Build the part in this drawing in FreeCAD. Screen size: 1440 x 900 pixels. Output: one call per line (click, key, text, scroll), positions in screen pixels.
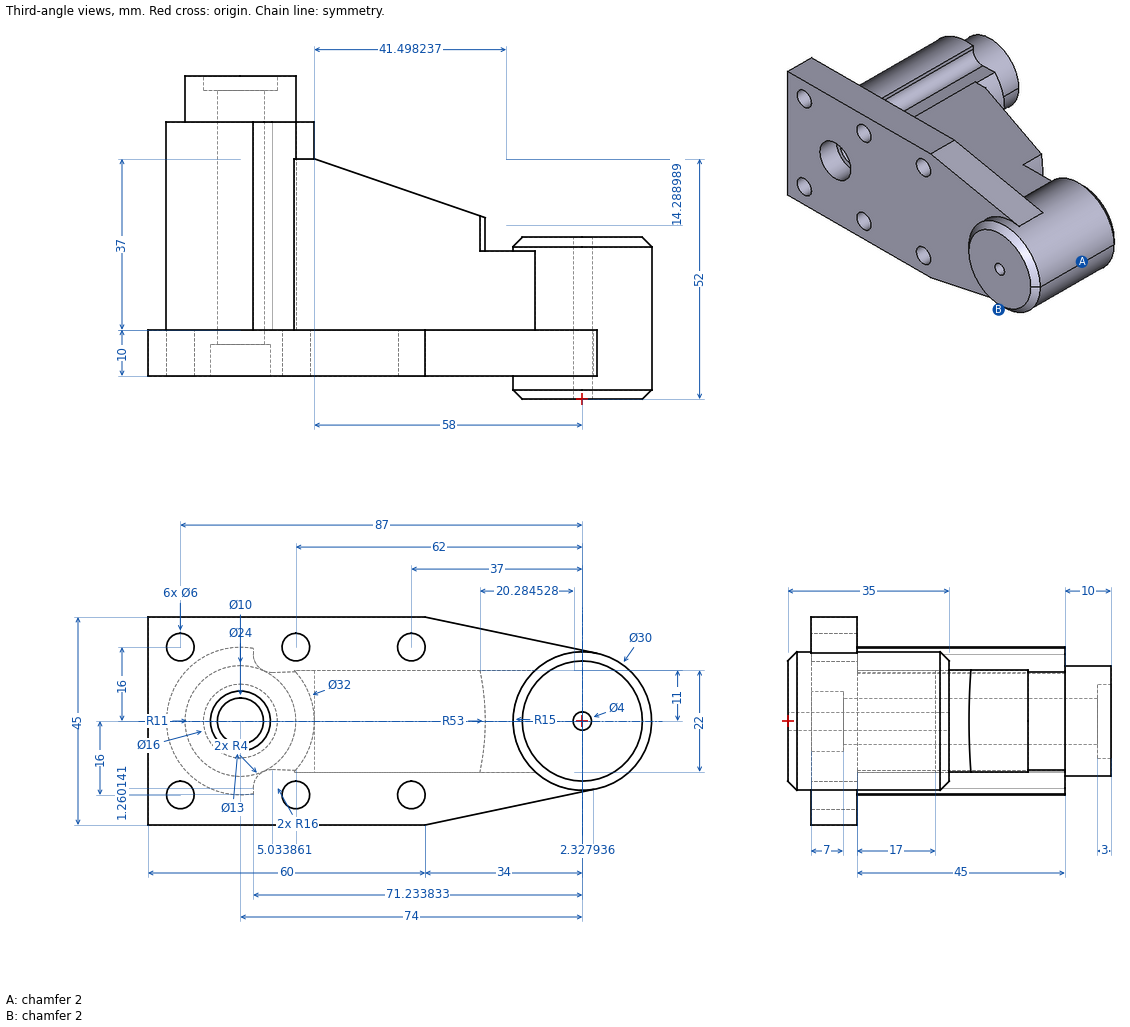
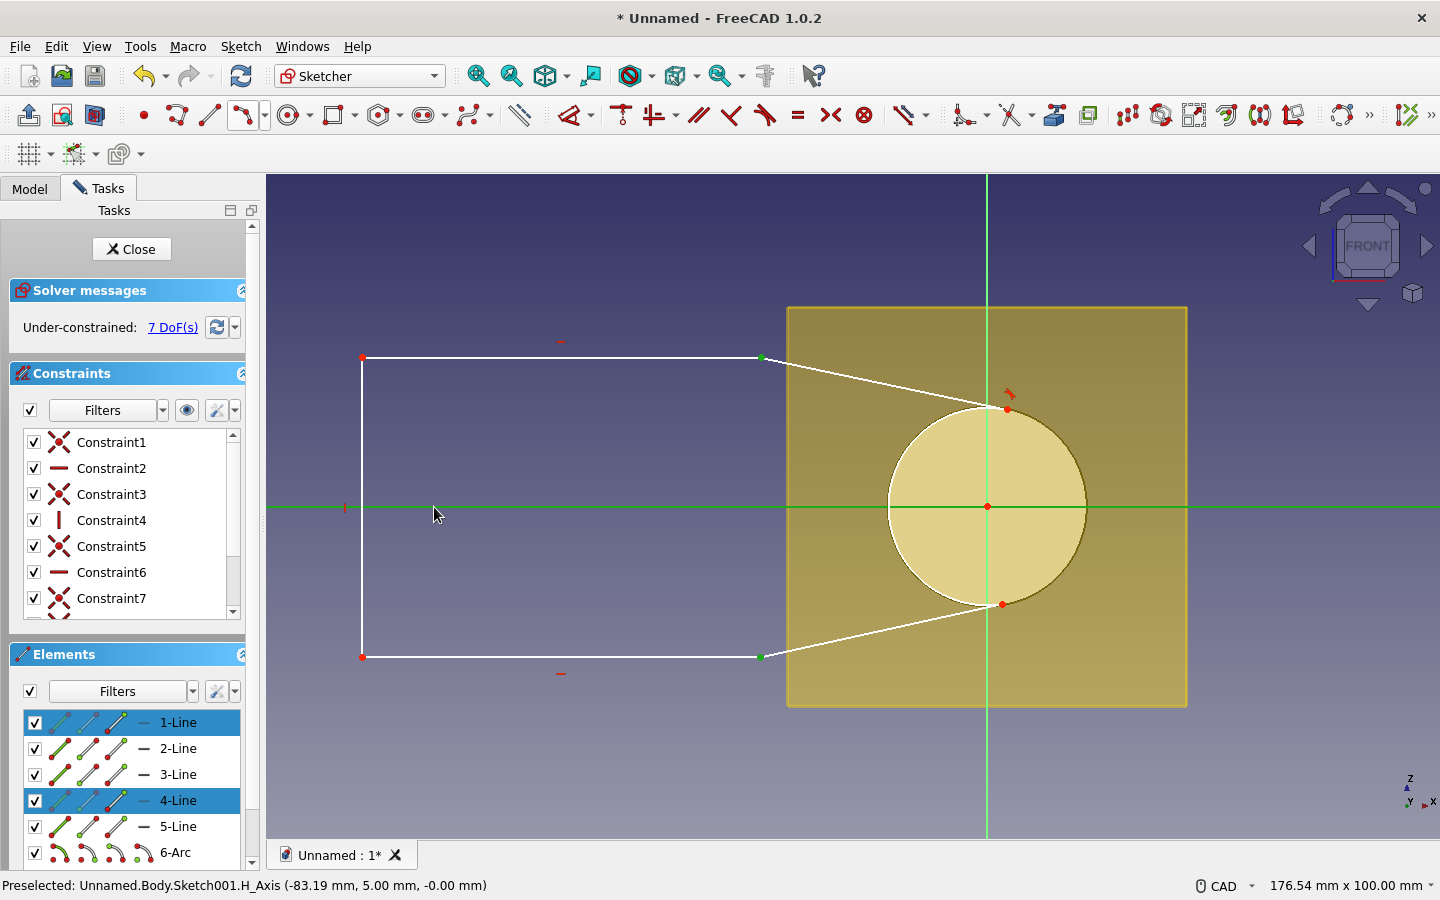
click(831, 116)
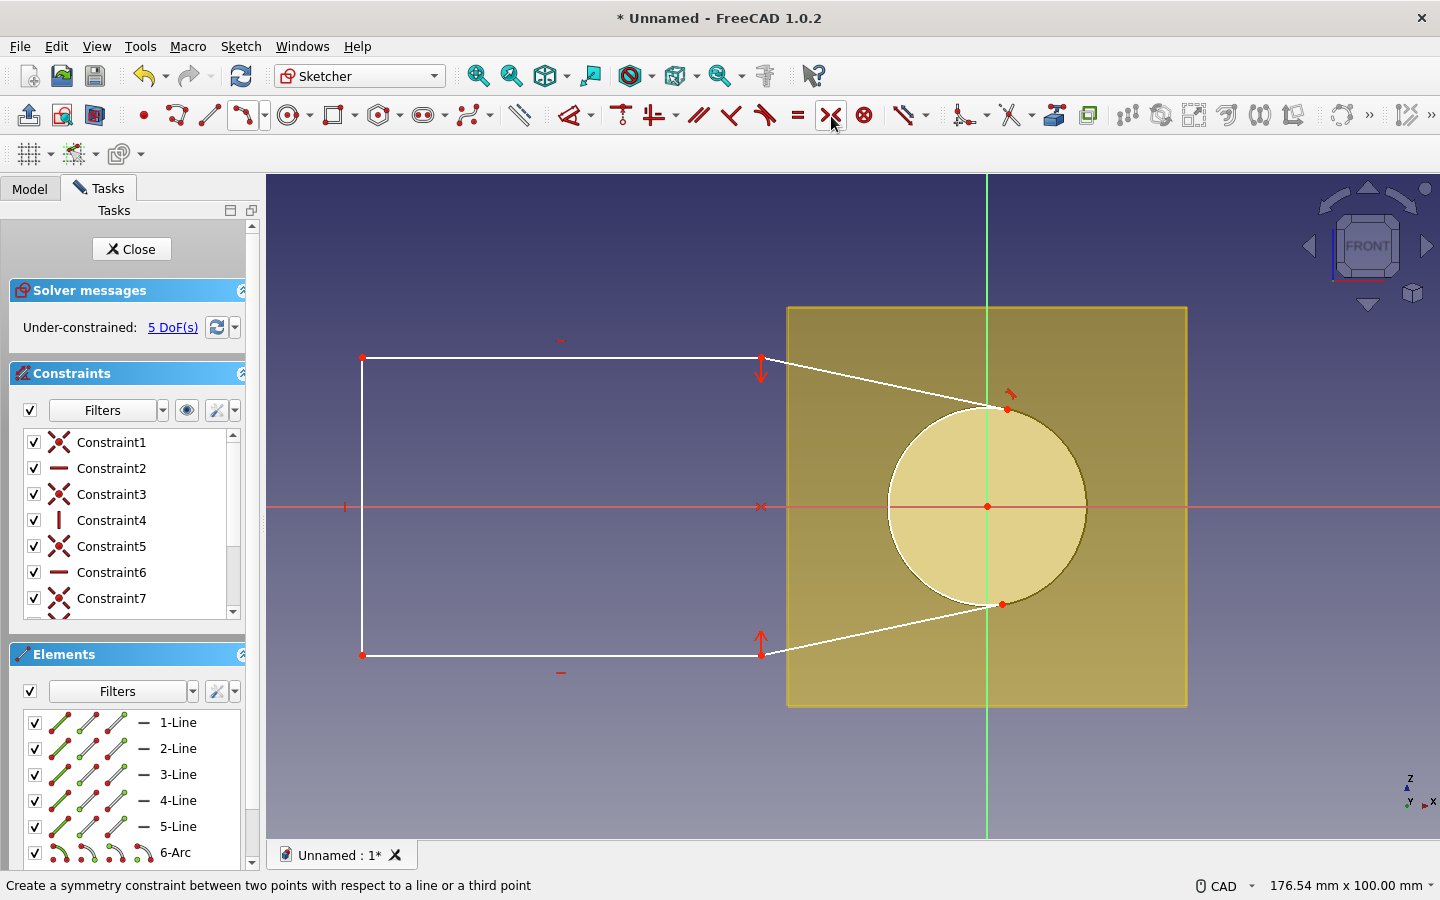
click(914, 441)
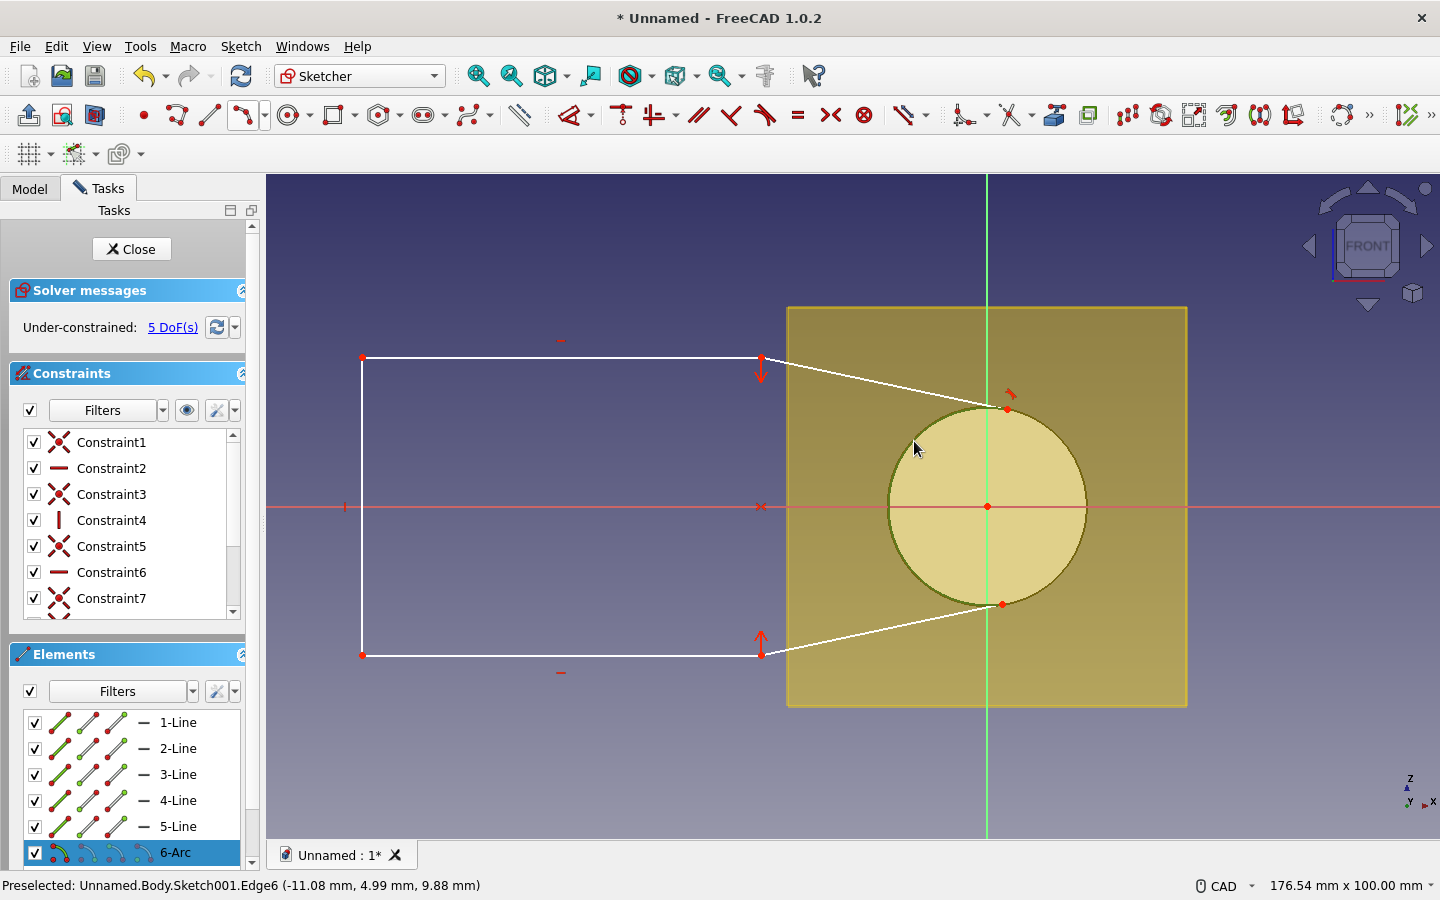
click(590, 116)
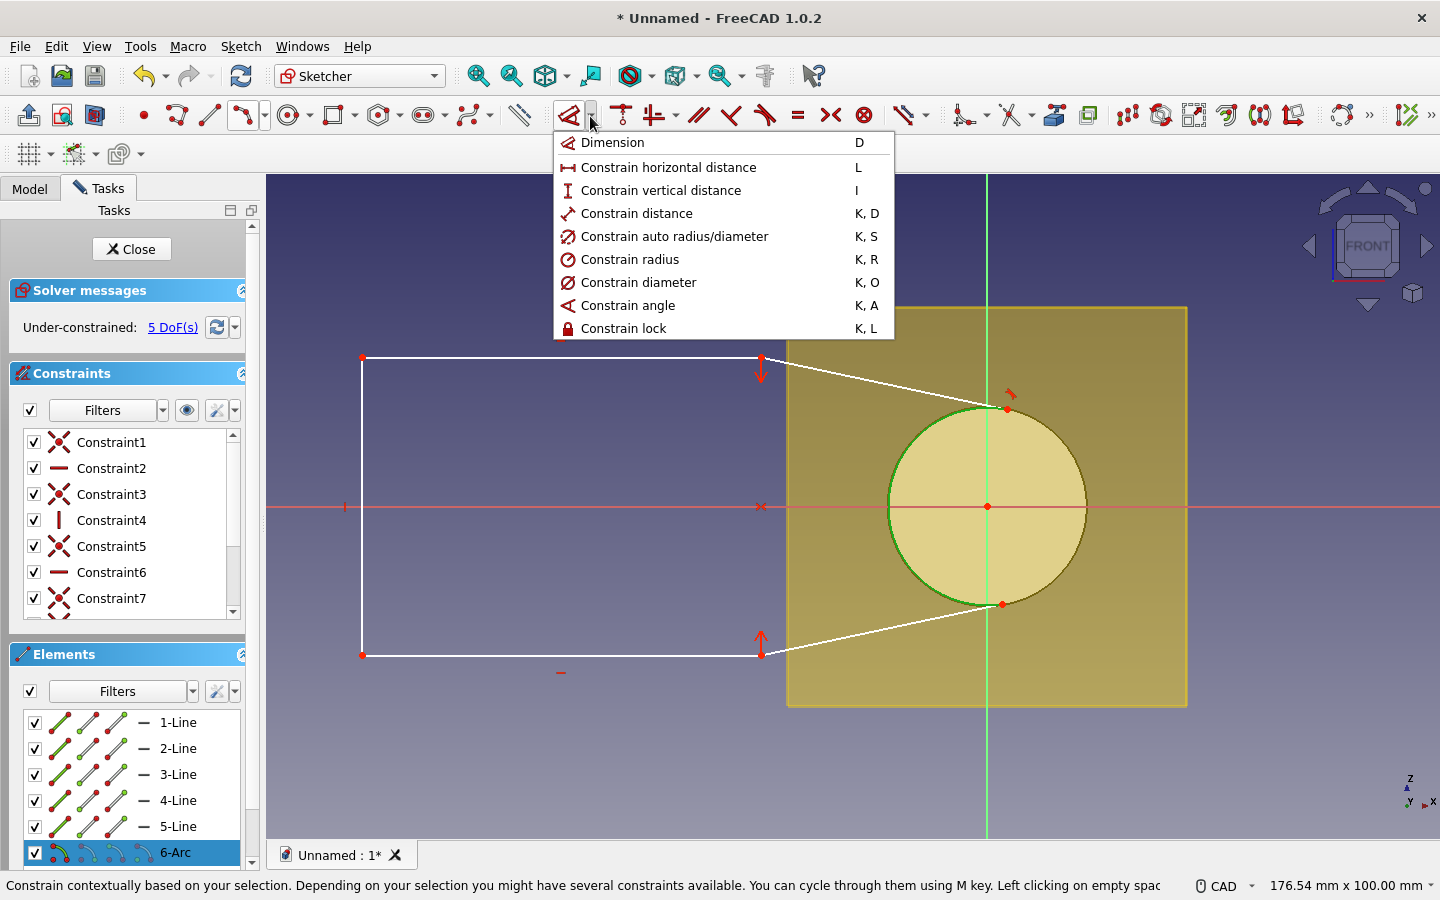
click(724, 260)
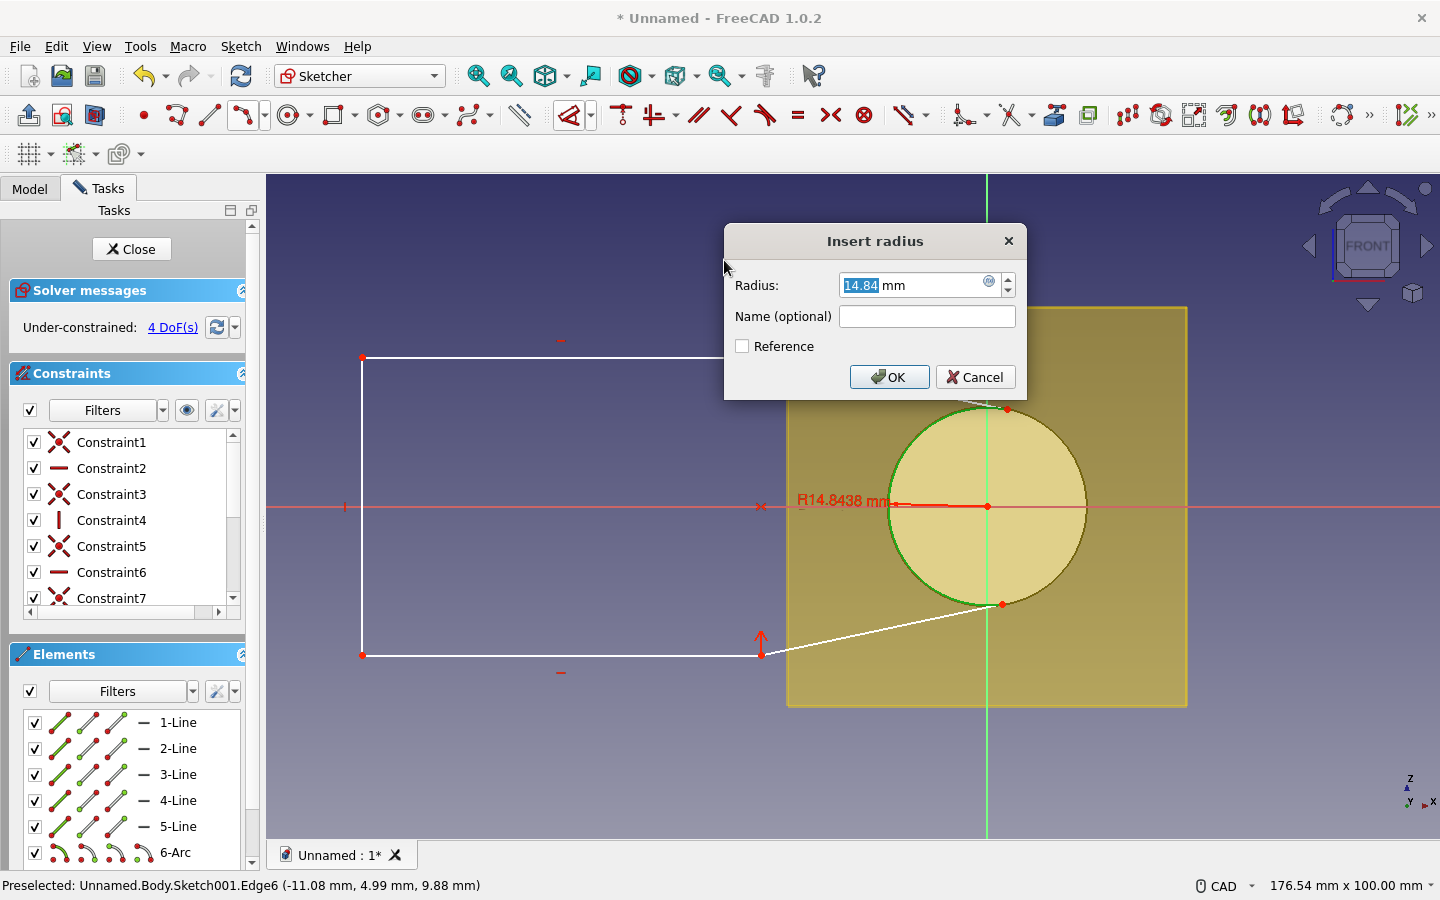
text(15)
key(Return)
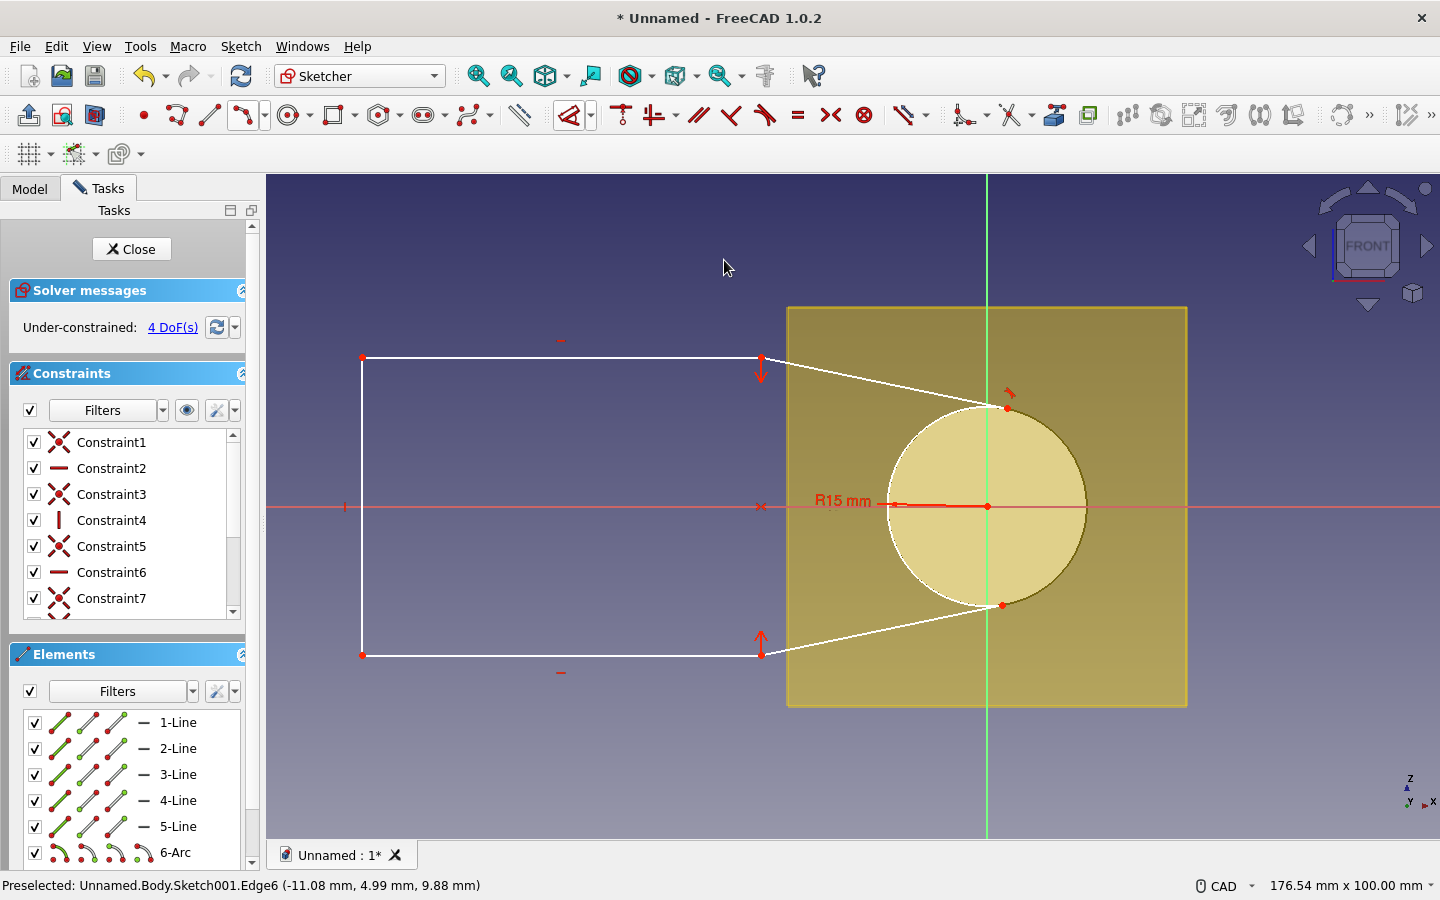
click(641, 656)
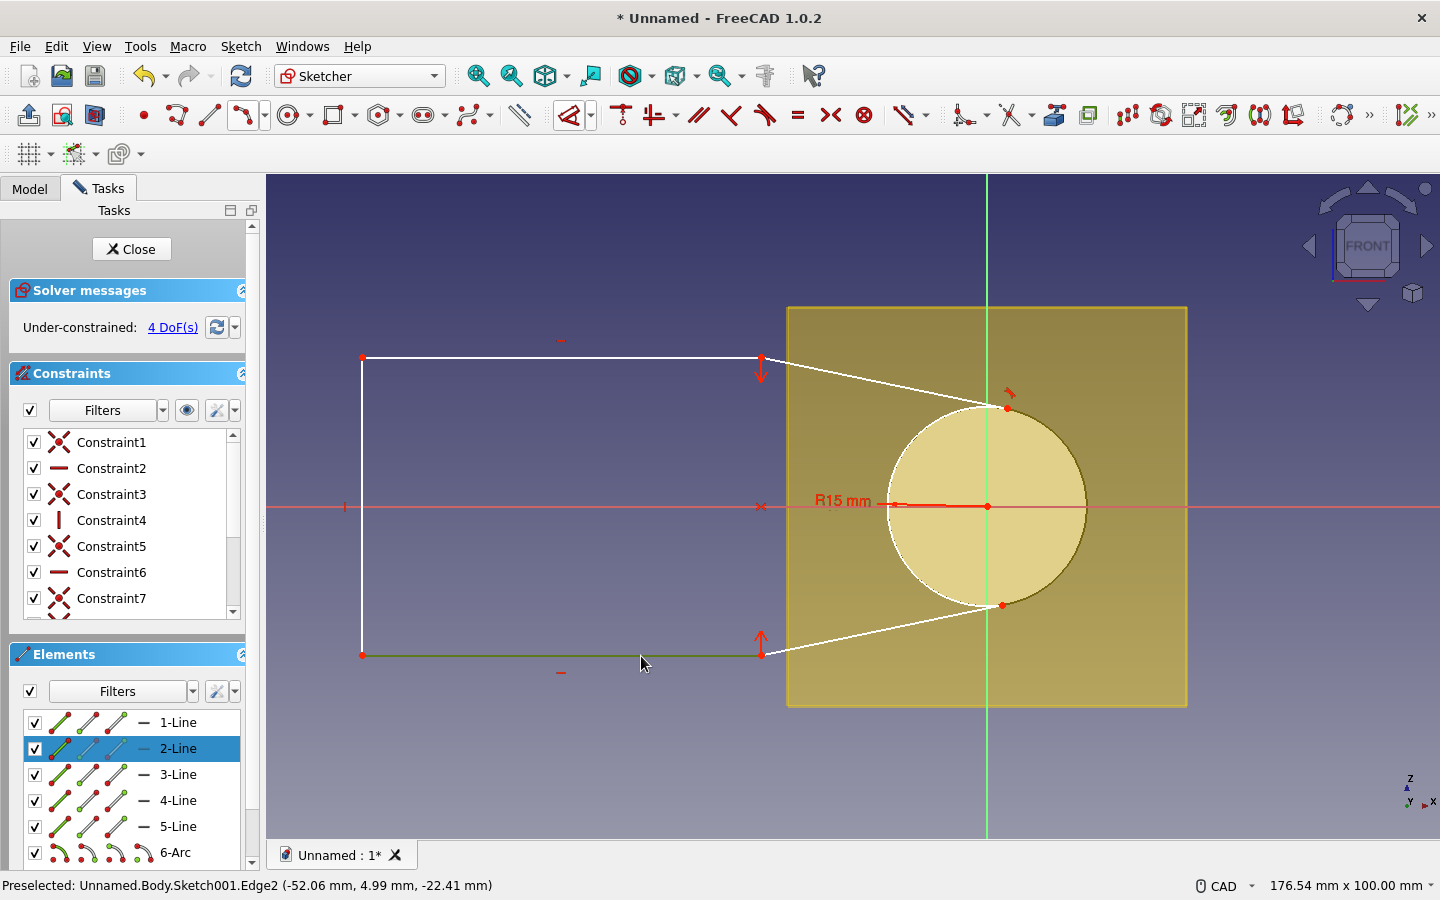
click(590, 116)